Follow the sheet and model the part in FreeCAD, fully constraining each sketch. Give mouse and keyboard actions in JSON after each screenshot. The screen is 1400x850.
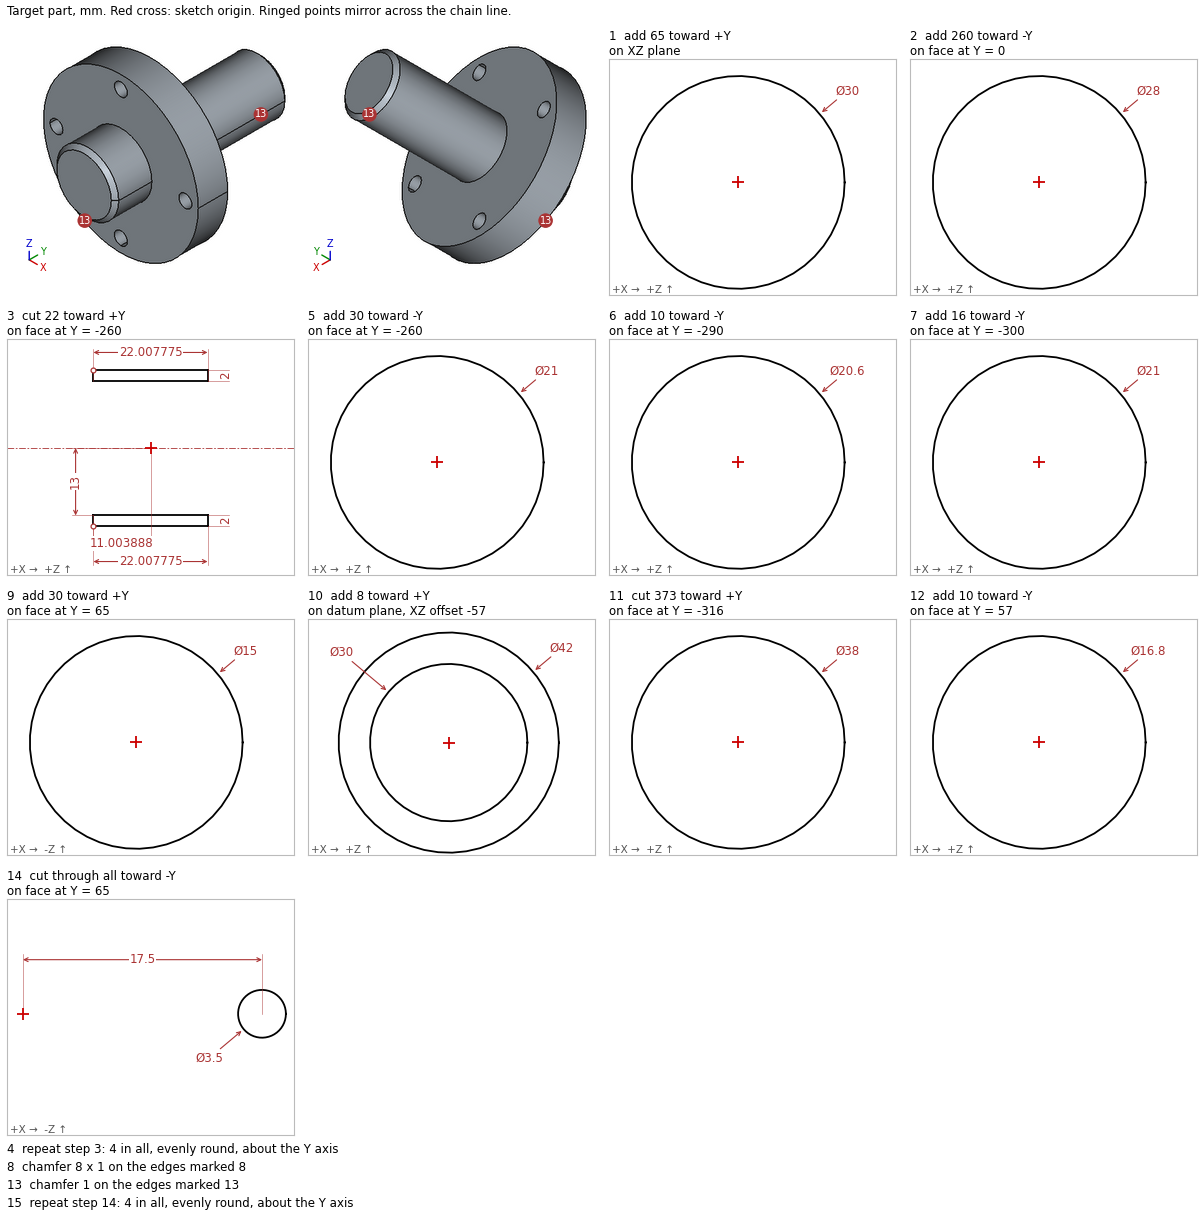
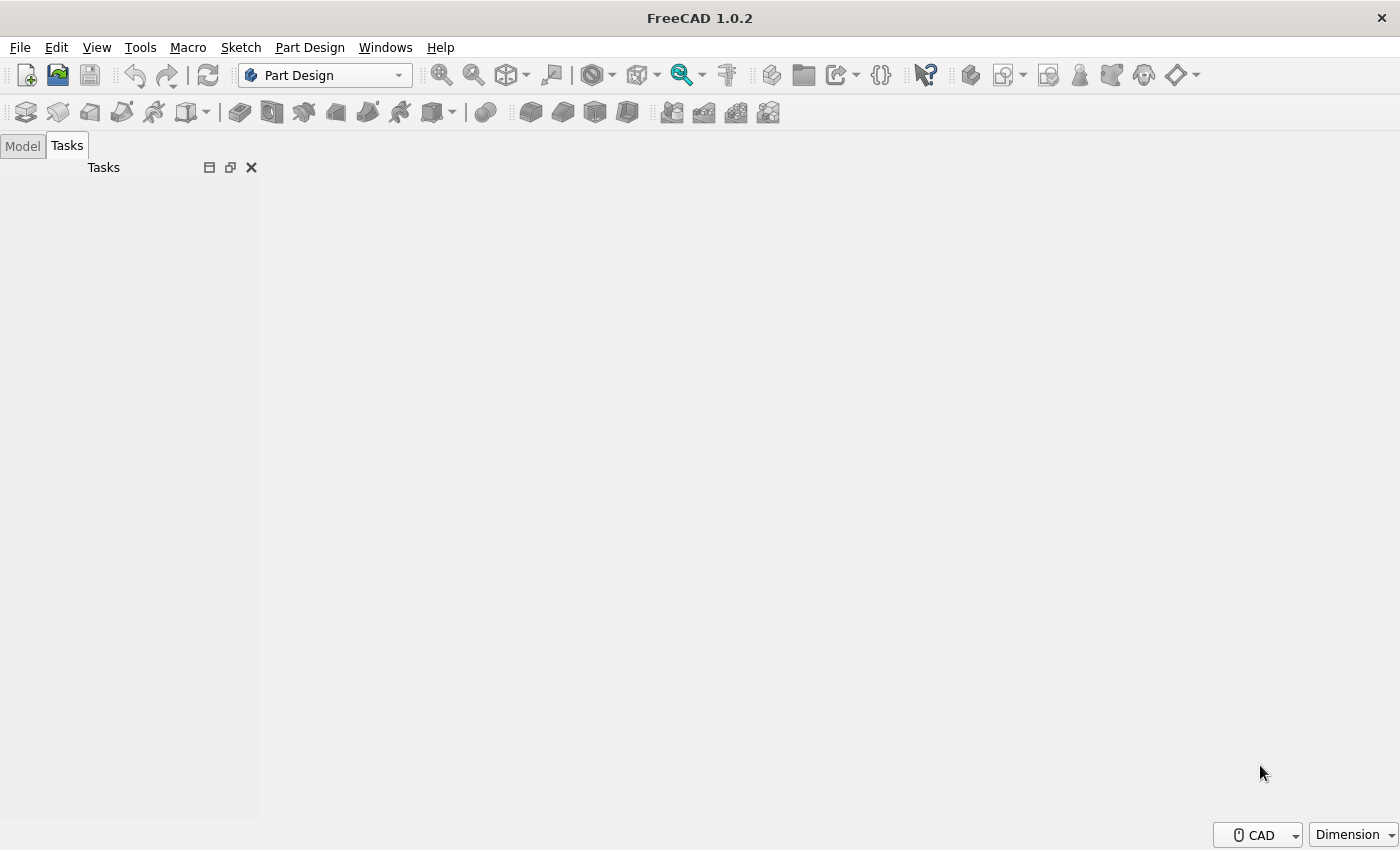
{"action": "key", "text": "ctrl+n"}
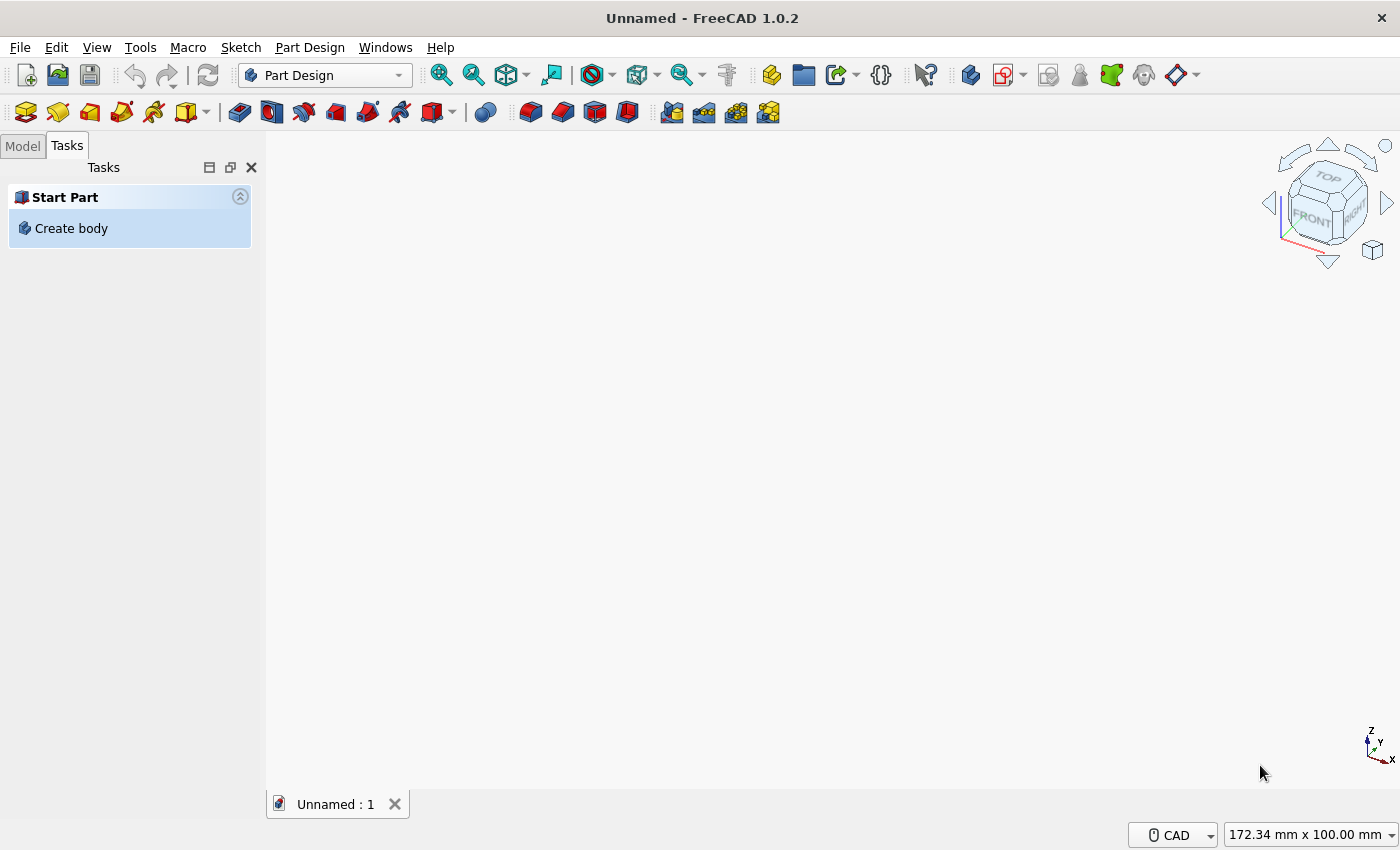
{"action": "left_click", "coordinate": [1004, 76]}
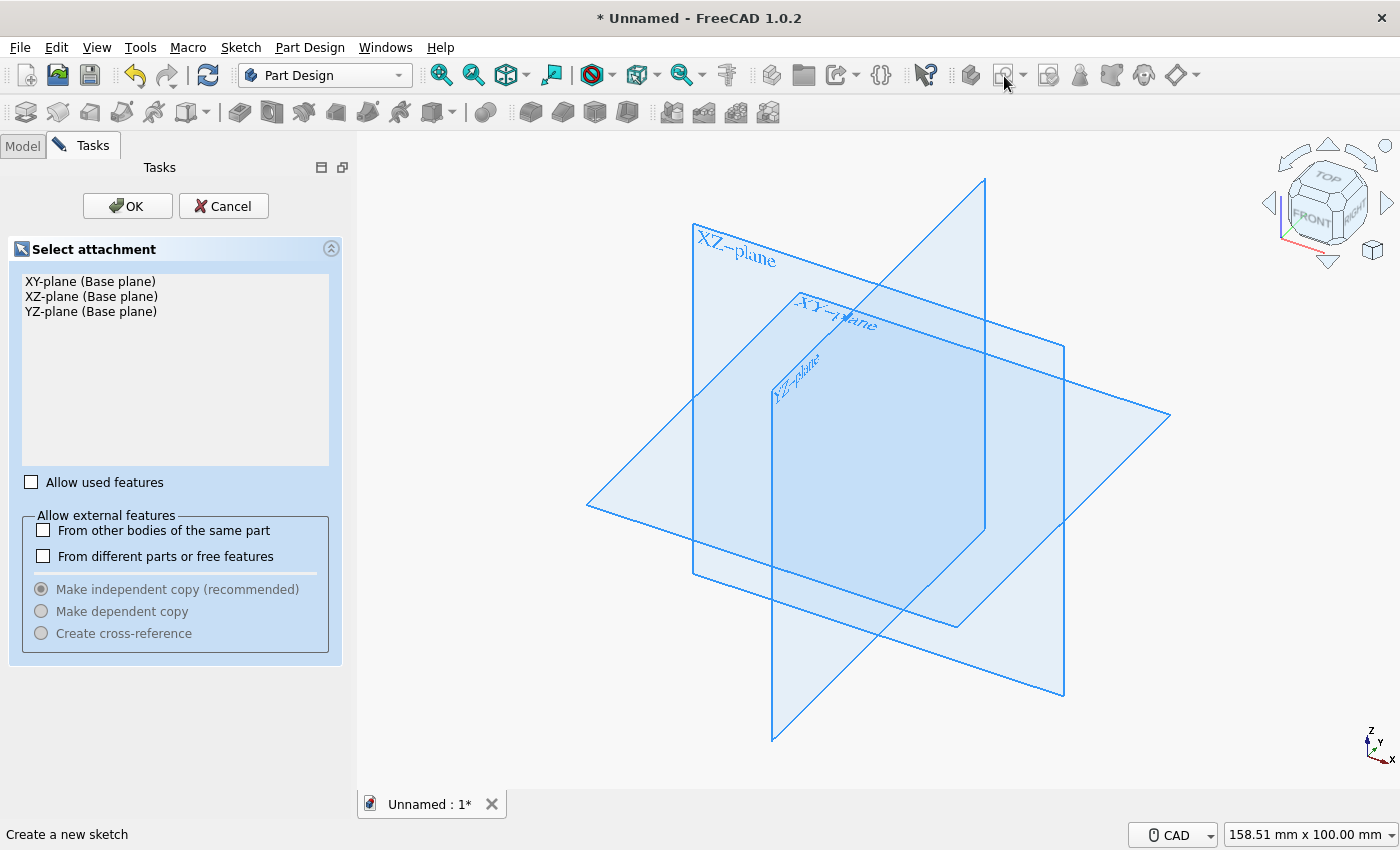
{"action": "left_click", "coordinate": [82, 296]}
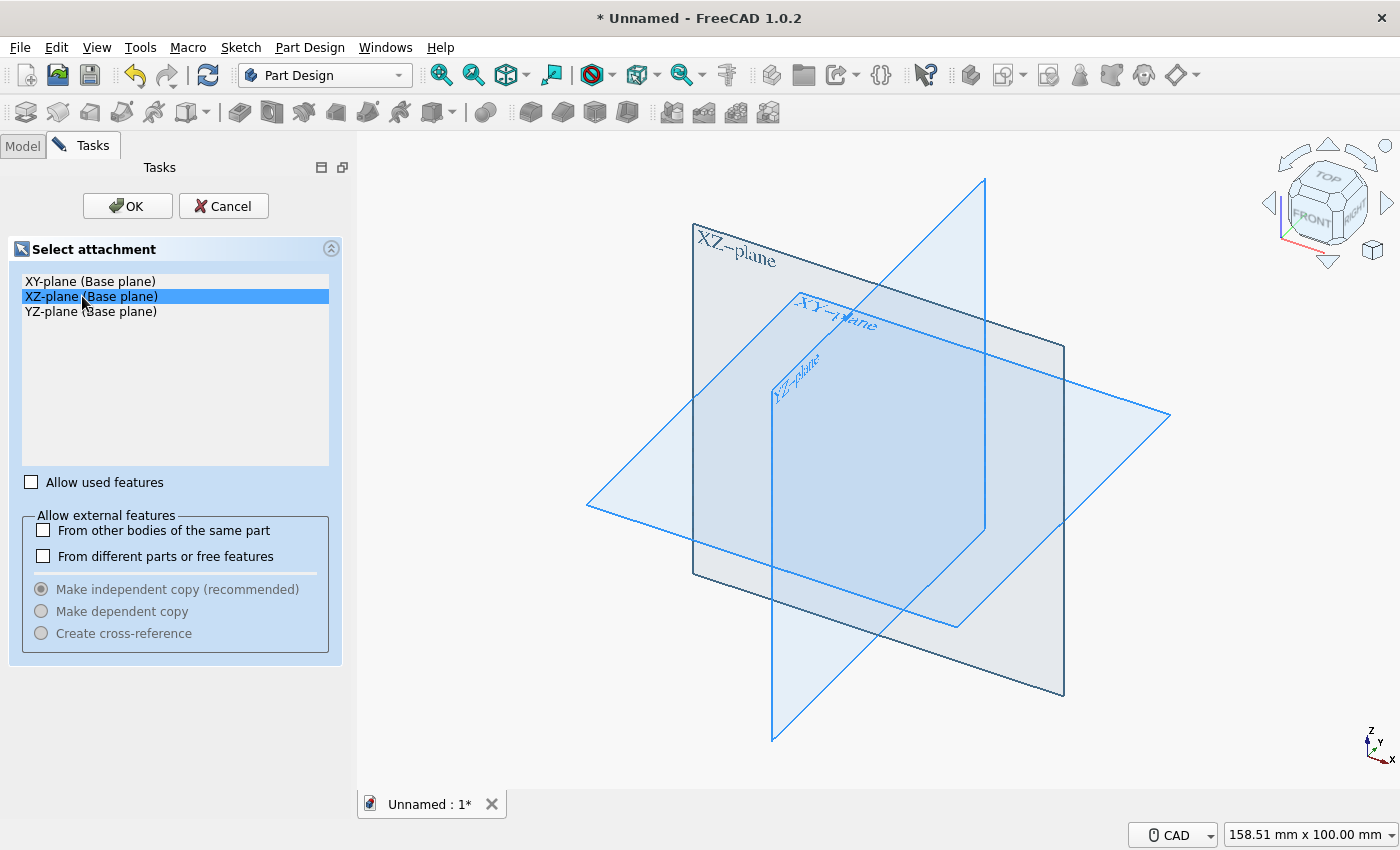
{"action": "left_click", "coordinate": [128, 206]}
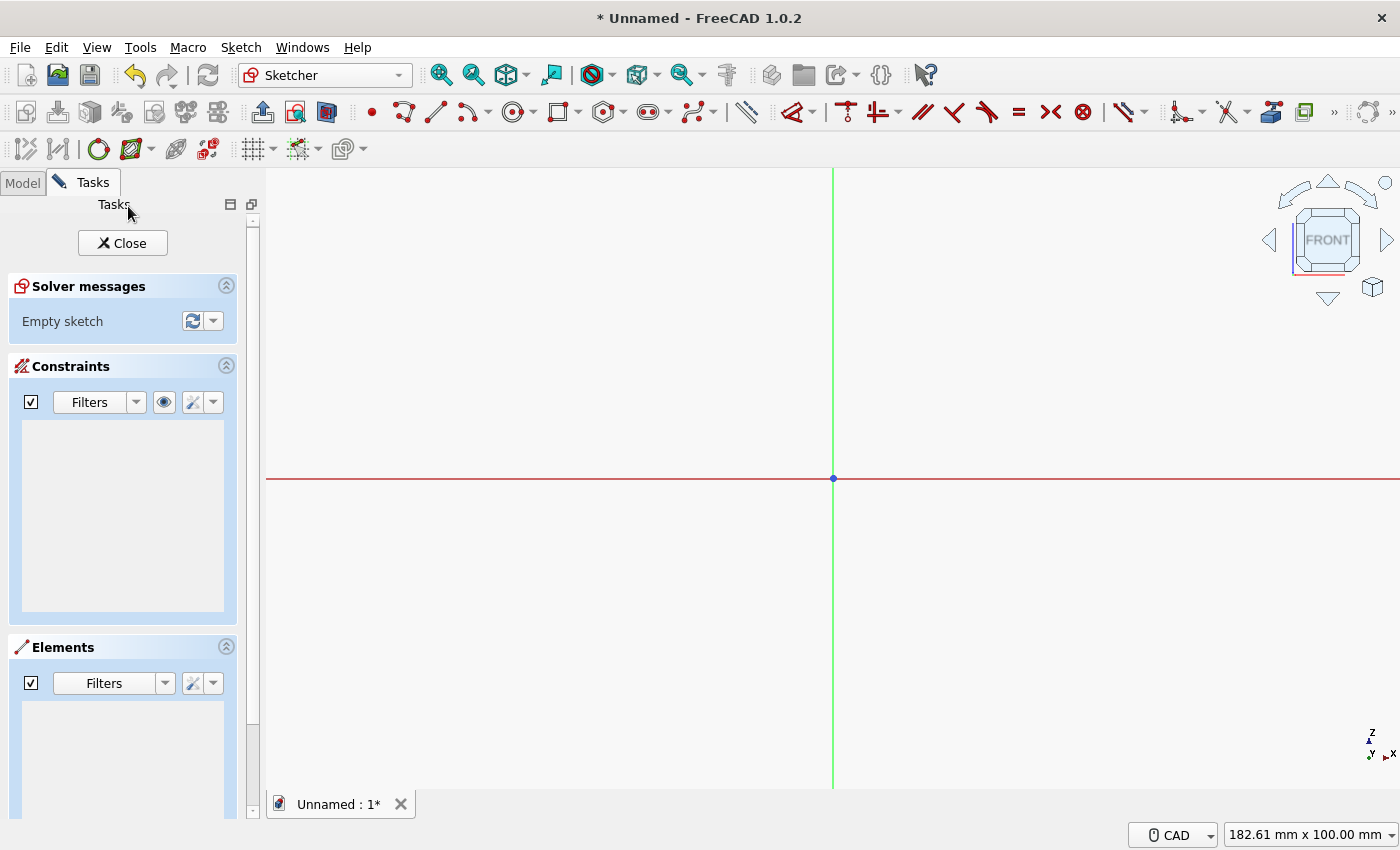
{"action": "scroll", "coordinate": [889, 478], "scroll_direction": "up", "scroll_amount": 4}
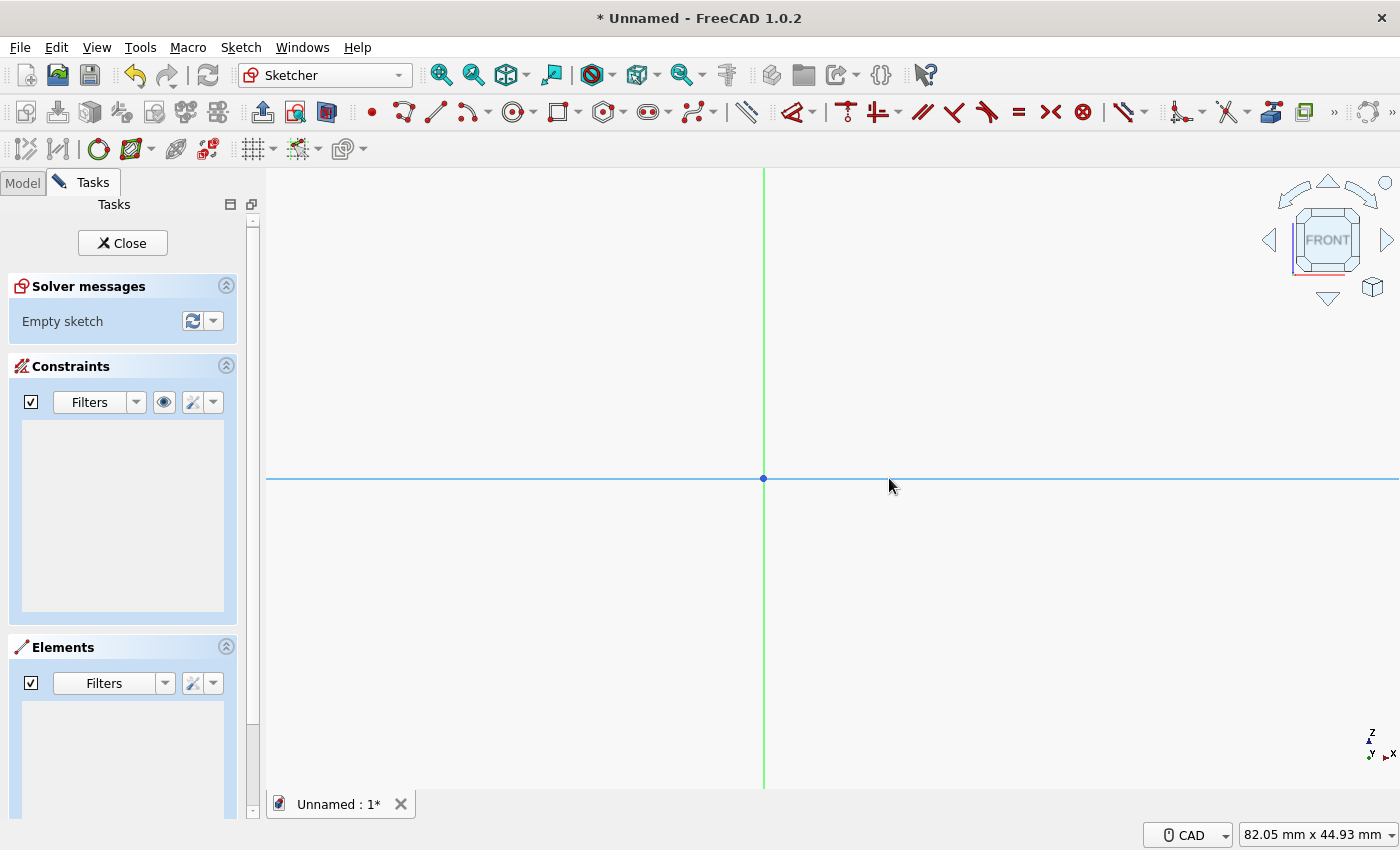
{"action": "left_click", "coordinate": [514, 112]}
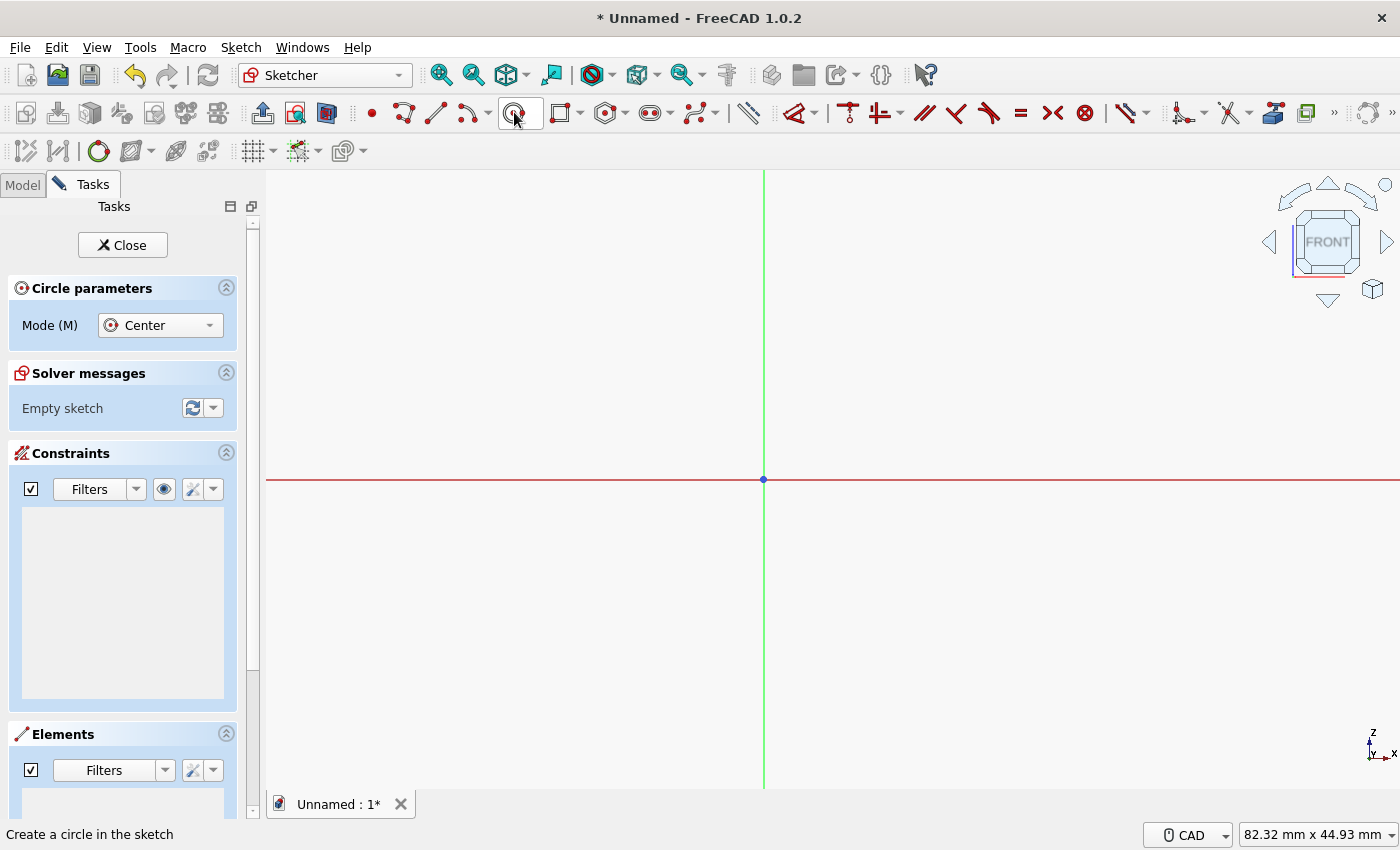
{"action": "left_click", "coordinate": [764, 480]}
{"action": "mouse_move", "coordinate": [910, 333]}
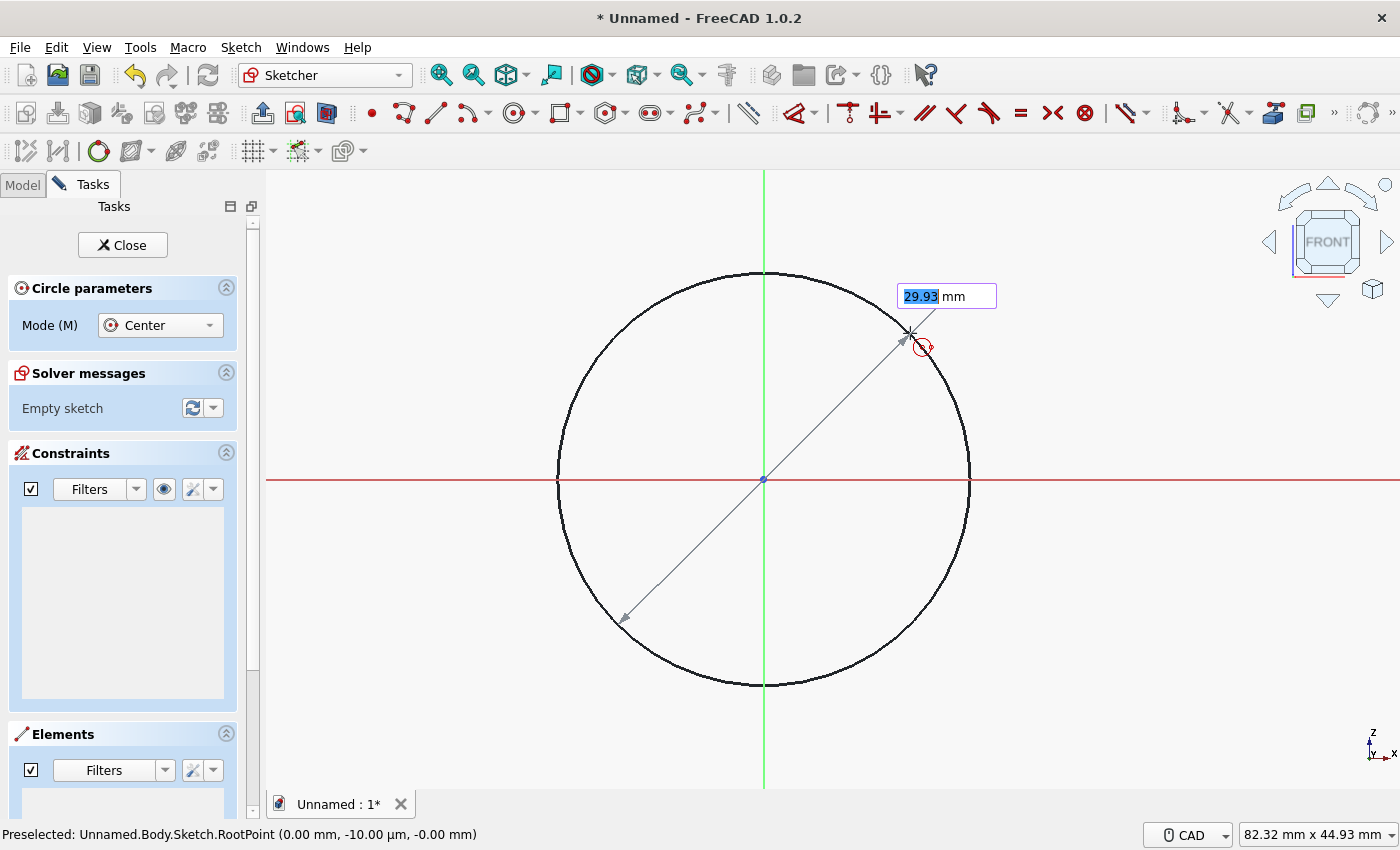
{"action": "type", "text": "30"}
{"action": "key", "text": "Return"}
{"action": "key", "text": "Escape"}